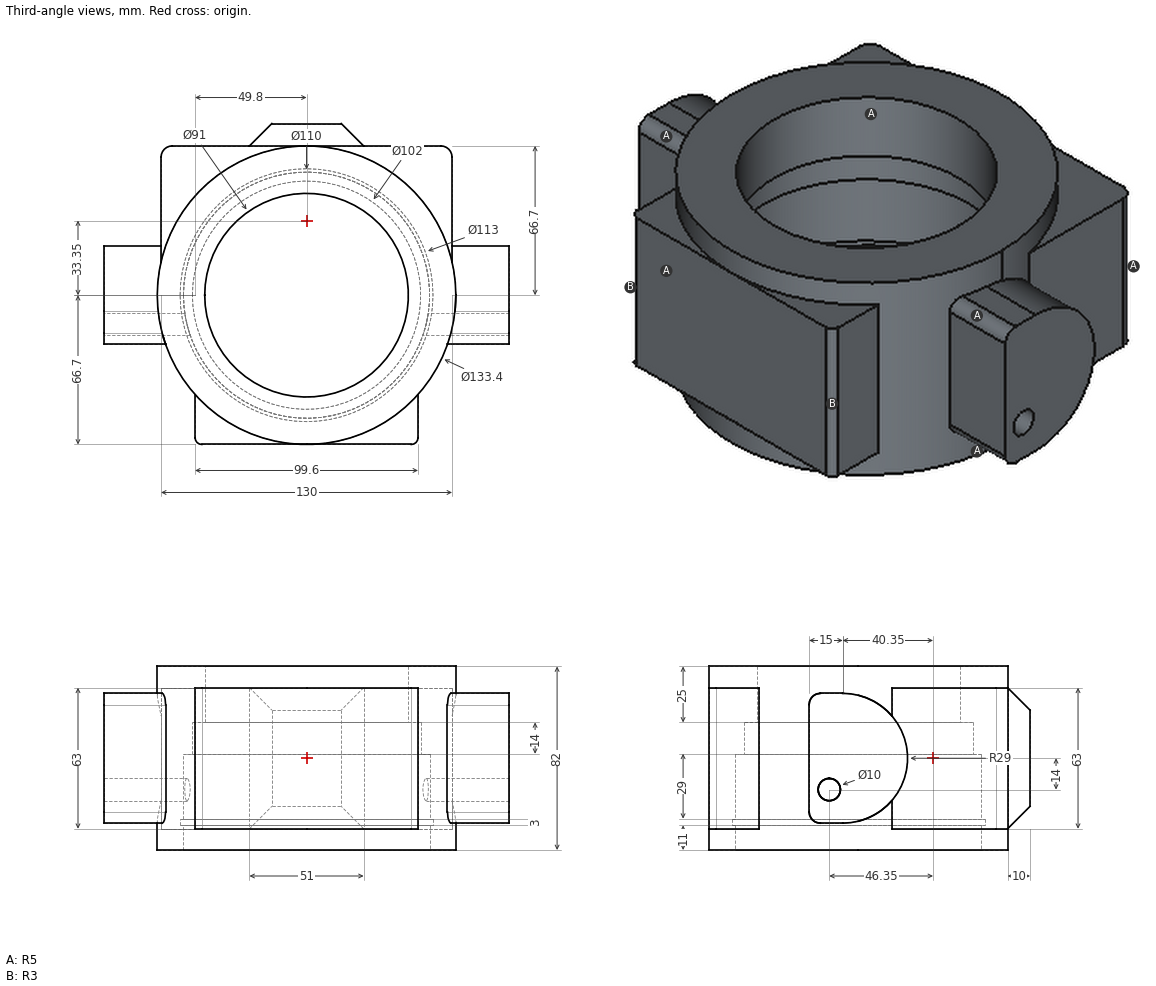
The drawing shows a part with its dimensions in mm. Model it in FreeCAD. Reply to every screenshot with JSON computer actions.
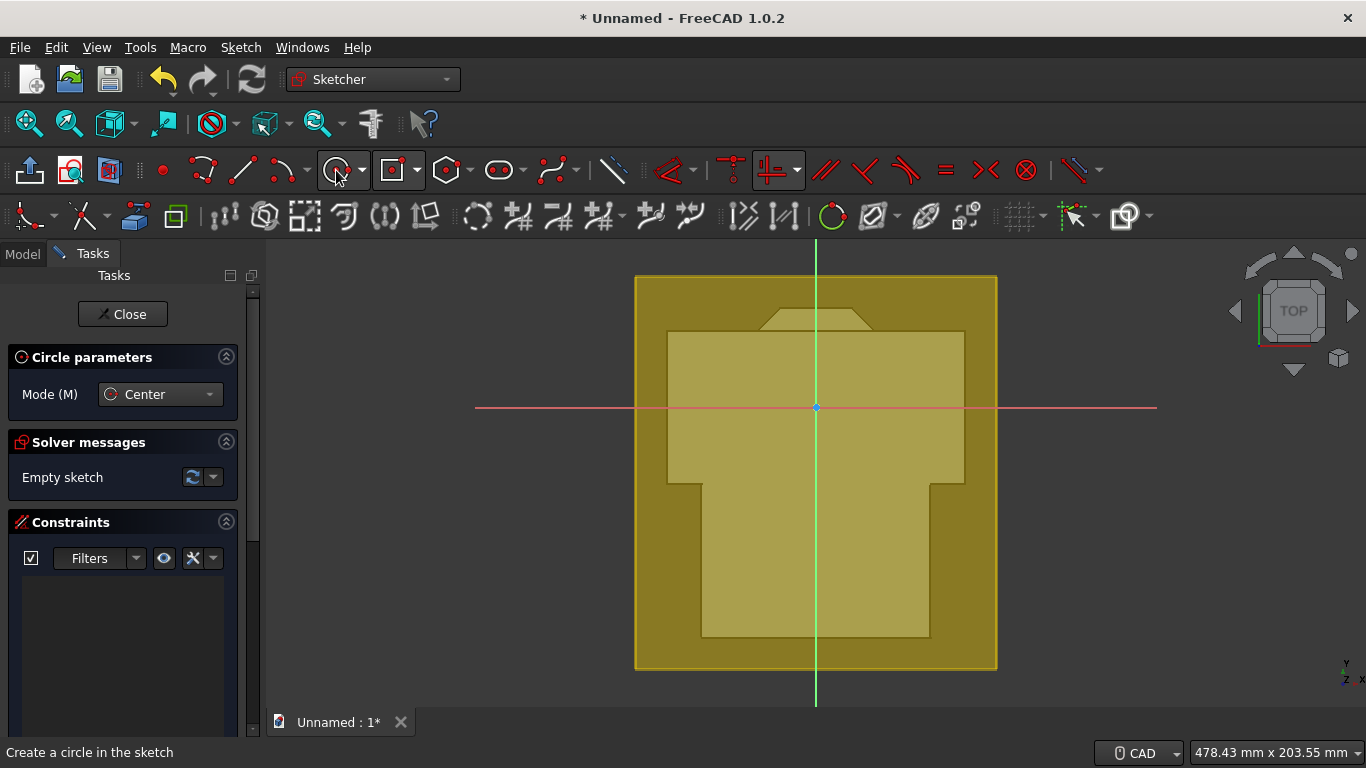
{"action": "left_click", "coordinate": [816, 484]}
{"action": "left_click", "coordinate": [924, 376]}
{"action": "key", "text": "Escape"}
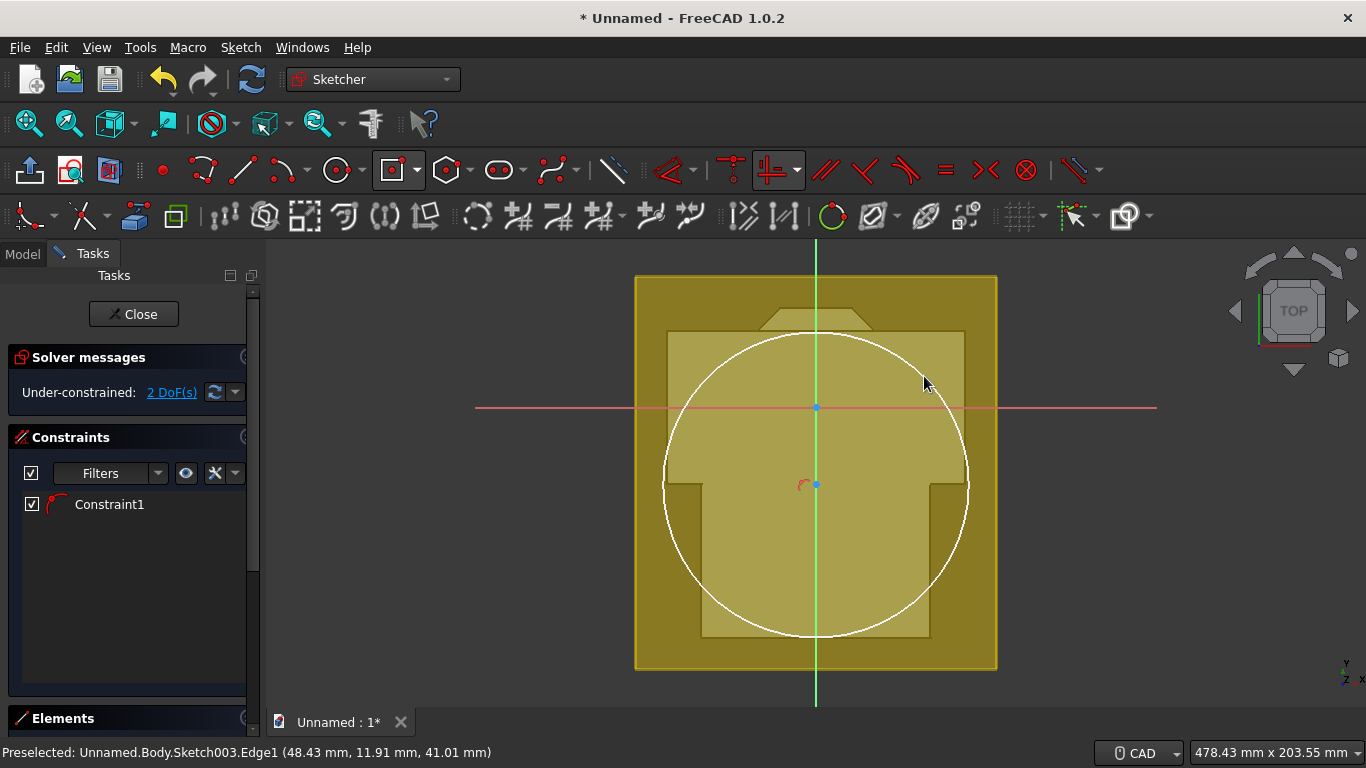
{"action": "key", "text": "d"}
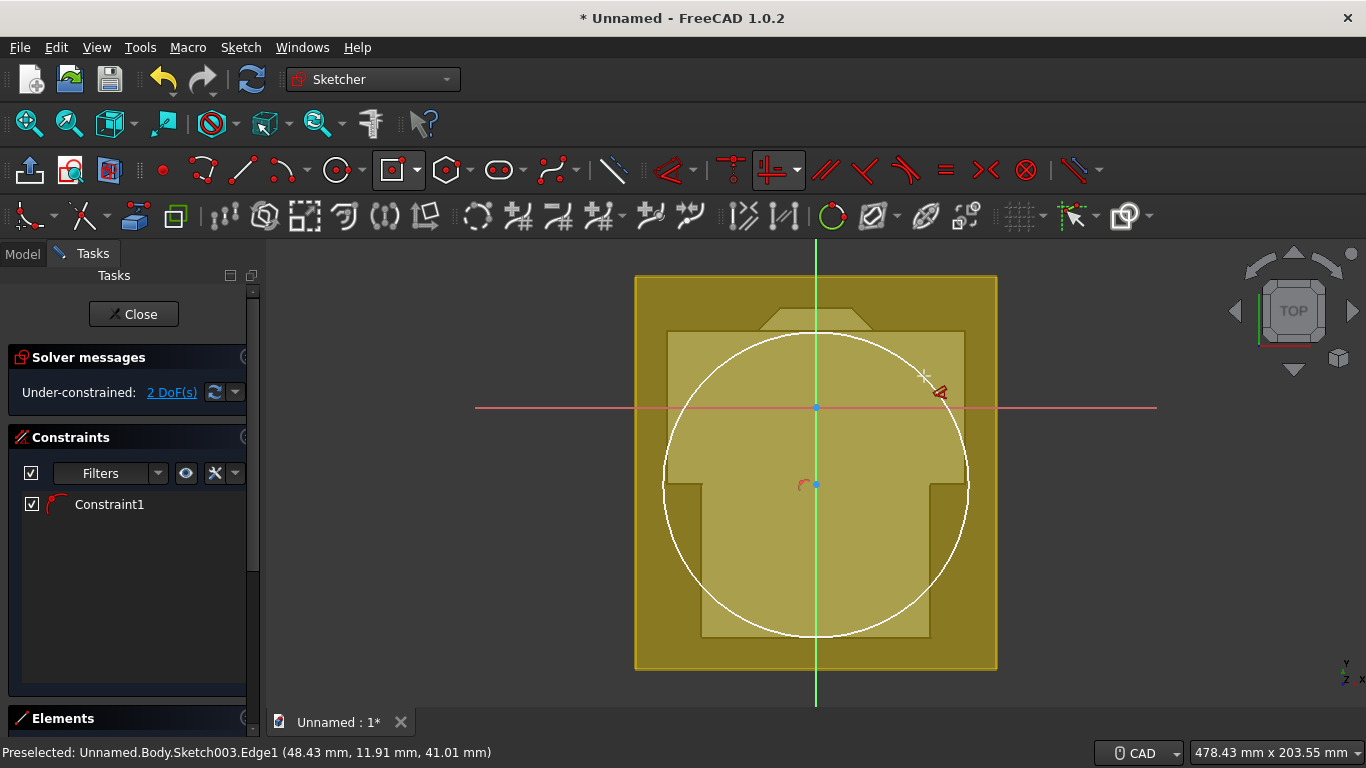
{"action": "left_click", "coordinate": [924, 377]}
{"action": "left_click", "coordinate": [947, 354]}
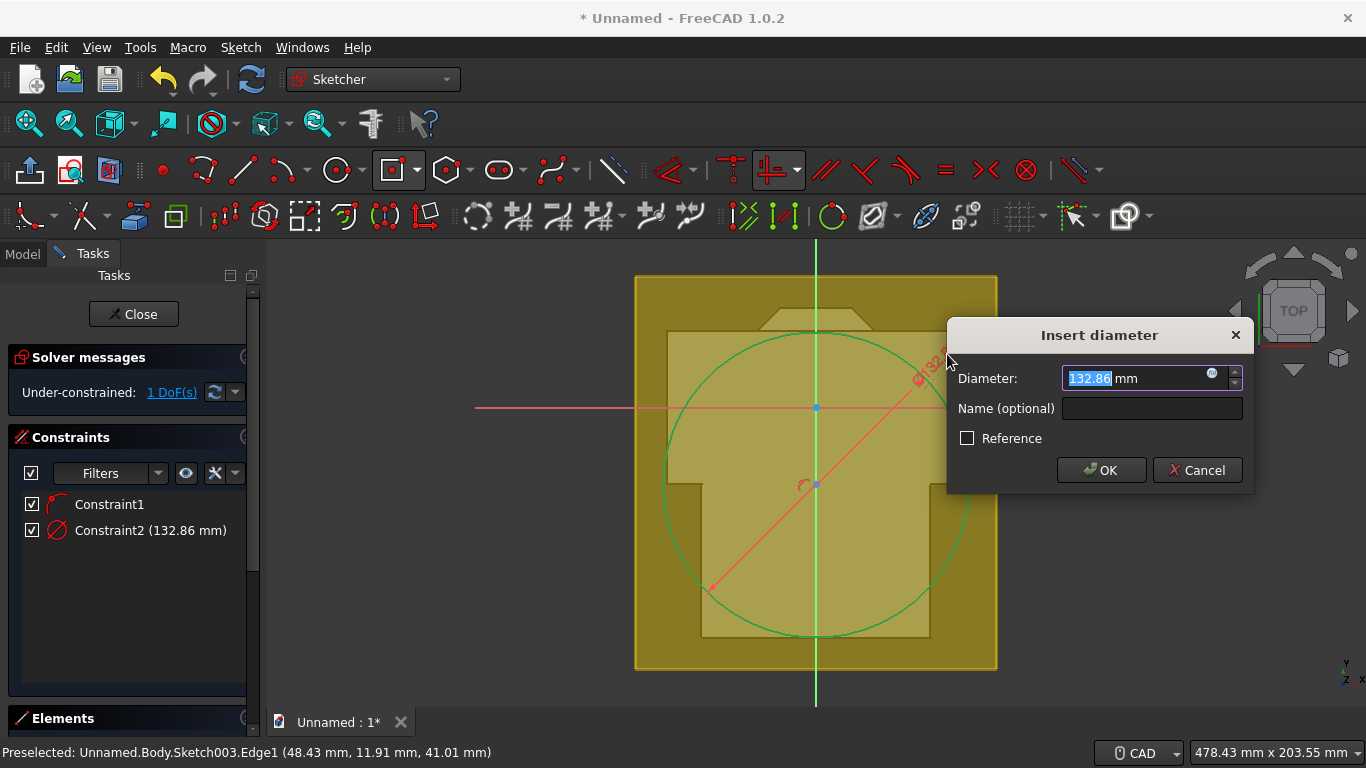
{"action": "type", "text": "133.4"}
{"action": "key", "text": "Return"}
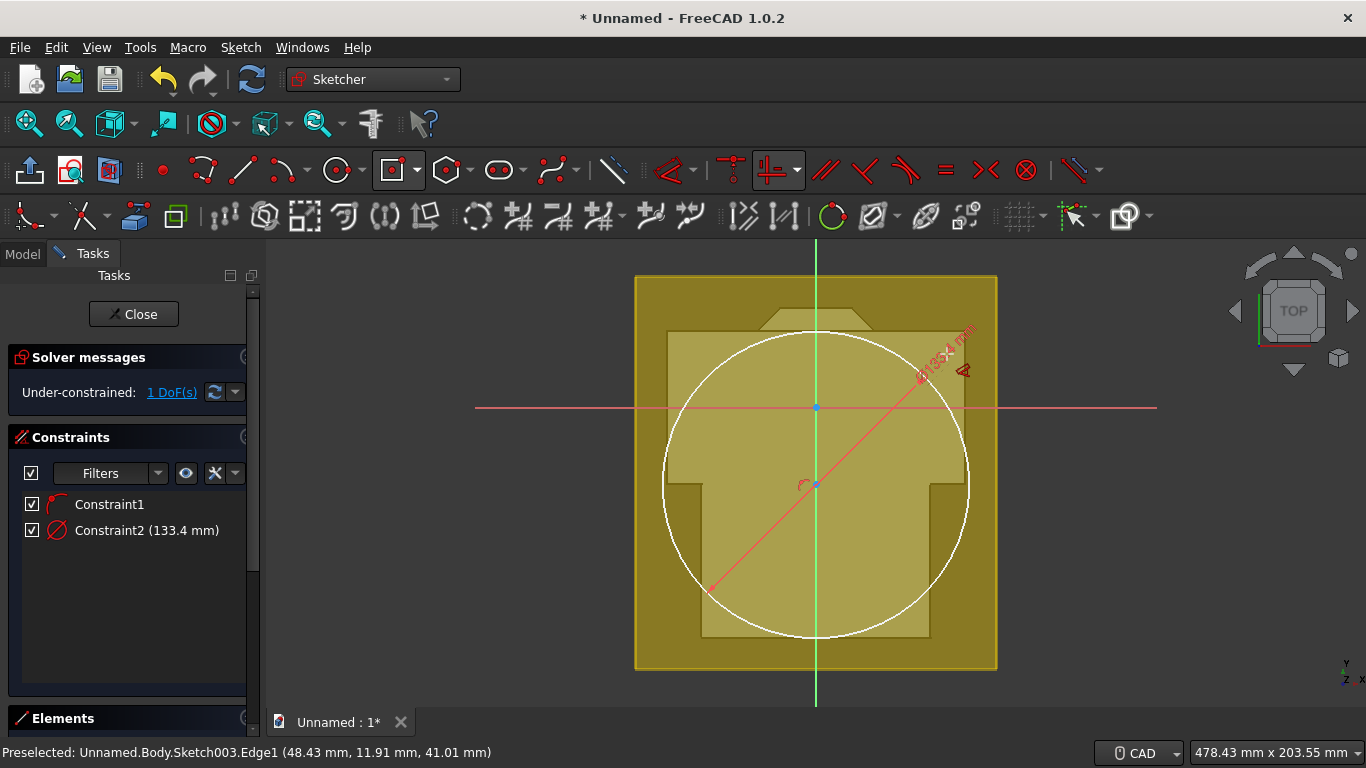
{"action": "left_click", "coordinate": [816, 485]}
{"action": "left_click", "coordinate": [850, 446]}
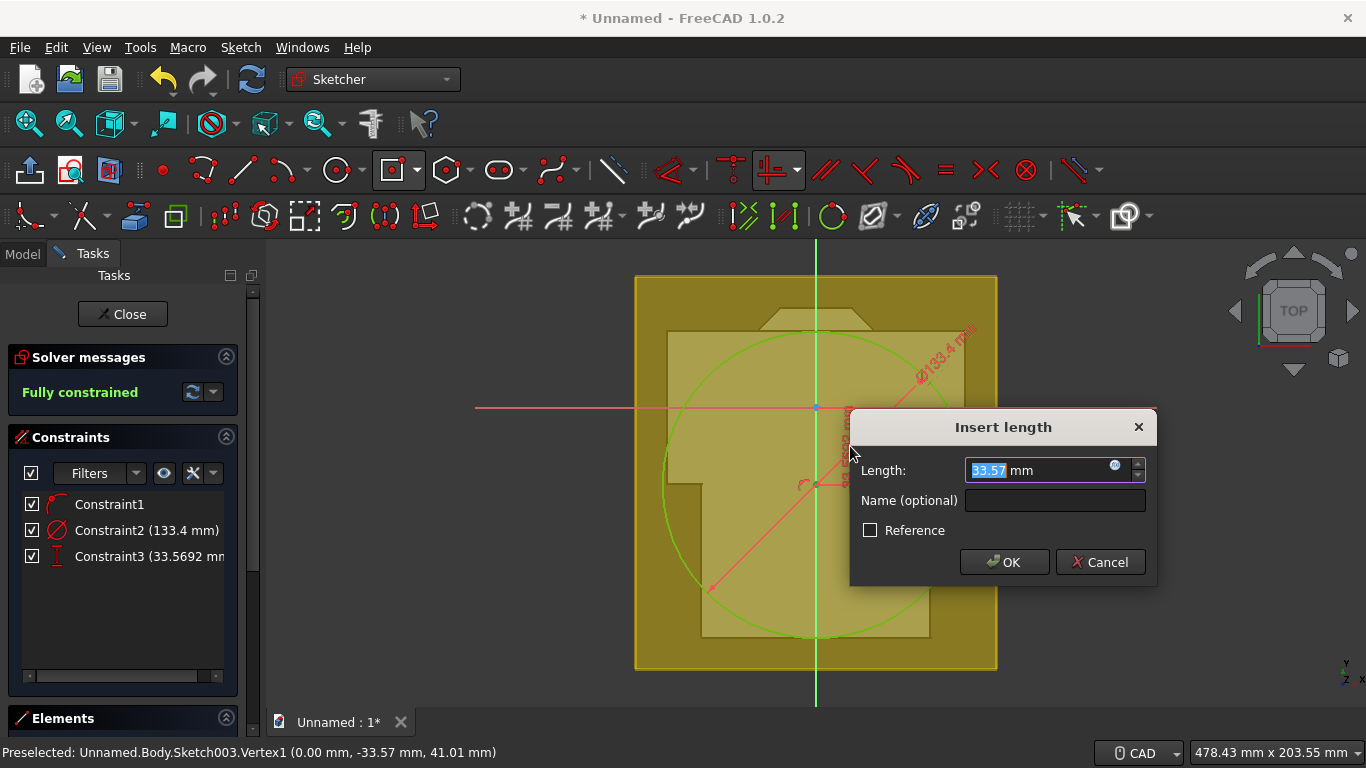
{"action": "type", "text": "33.35"}
{"action": "key", "text": "Return"}
{"action": "key", "text": "Escape"}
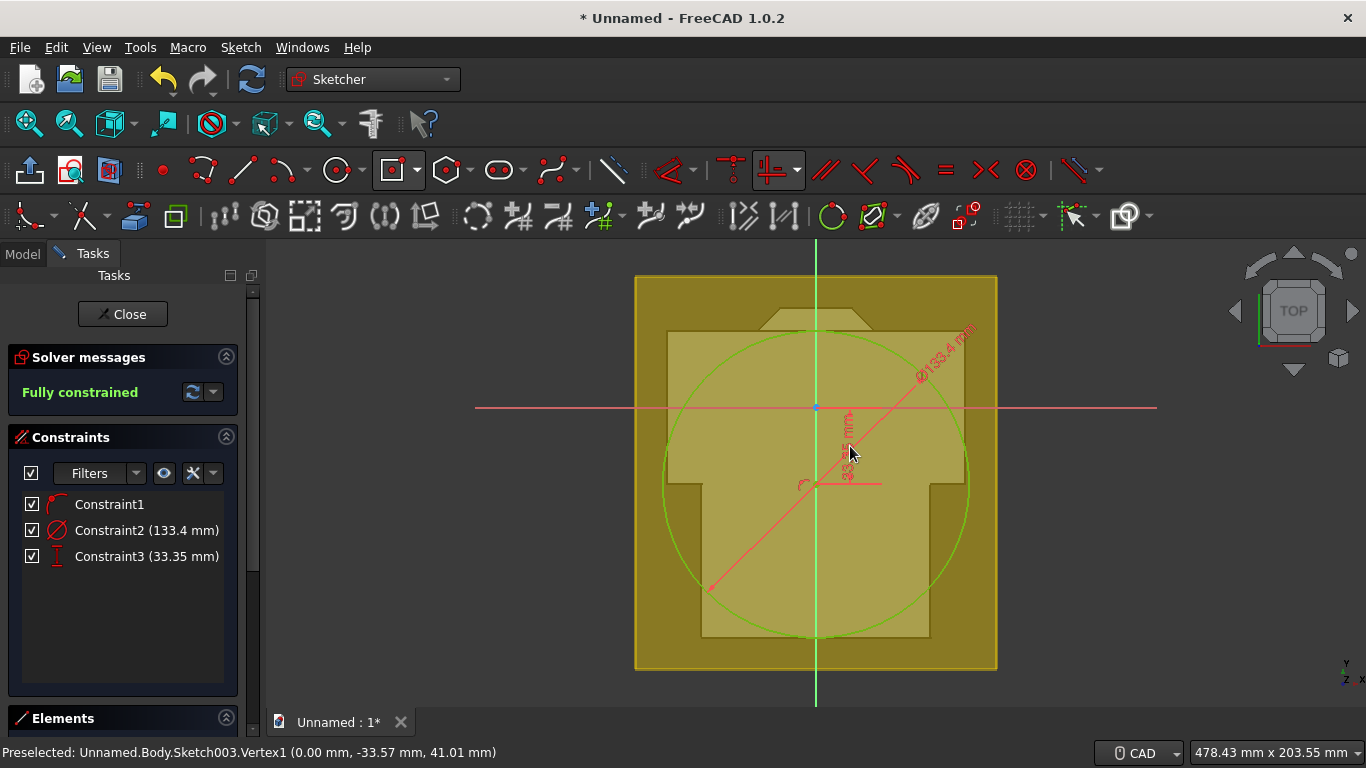
{"action": "left_click", "coordinate": [123, 314]}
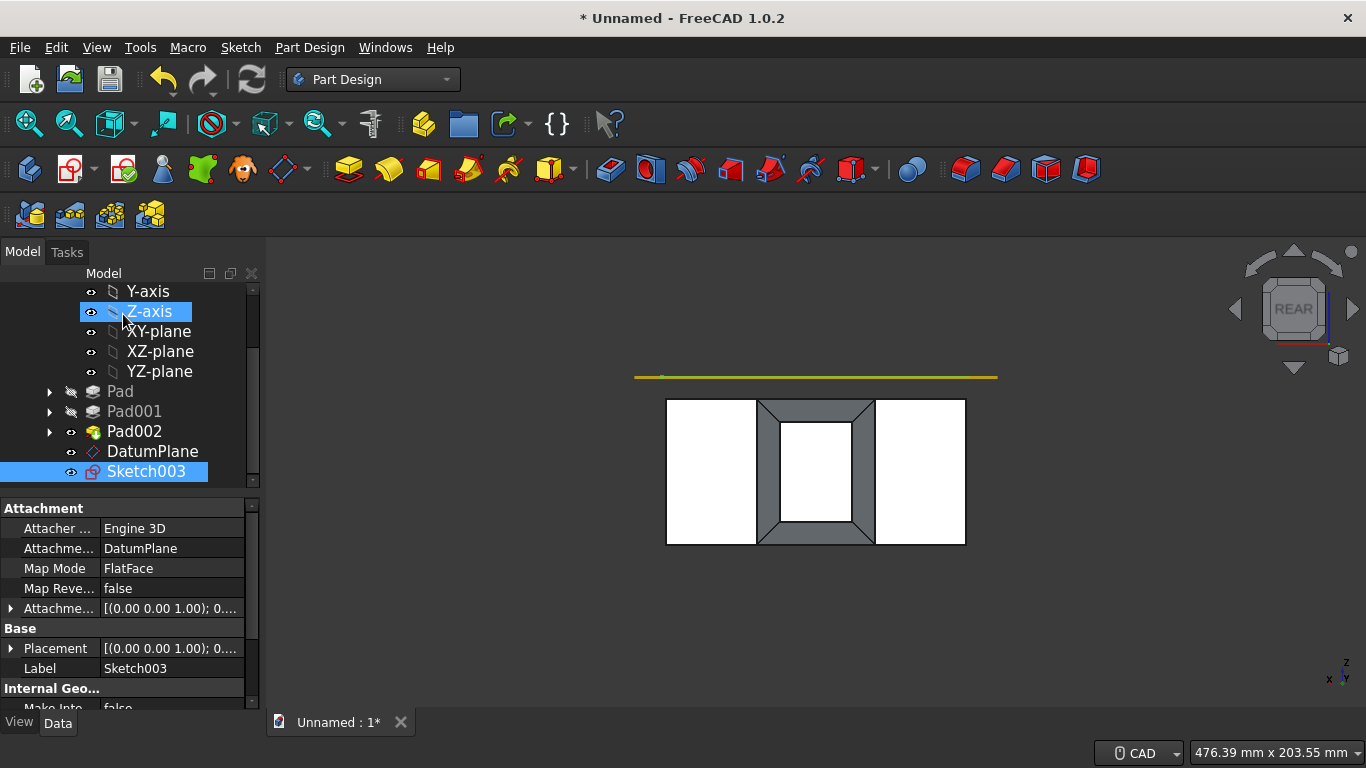
{"action": "left_click", "coordinate": [350, 170]}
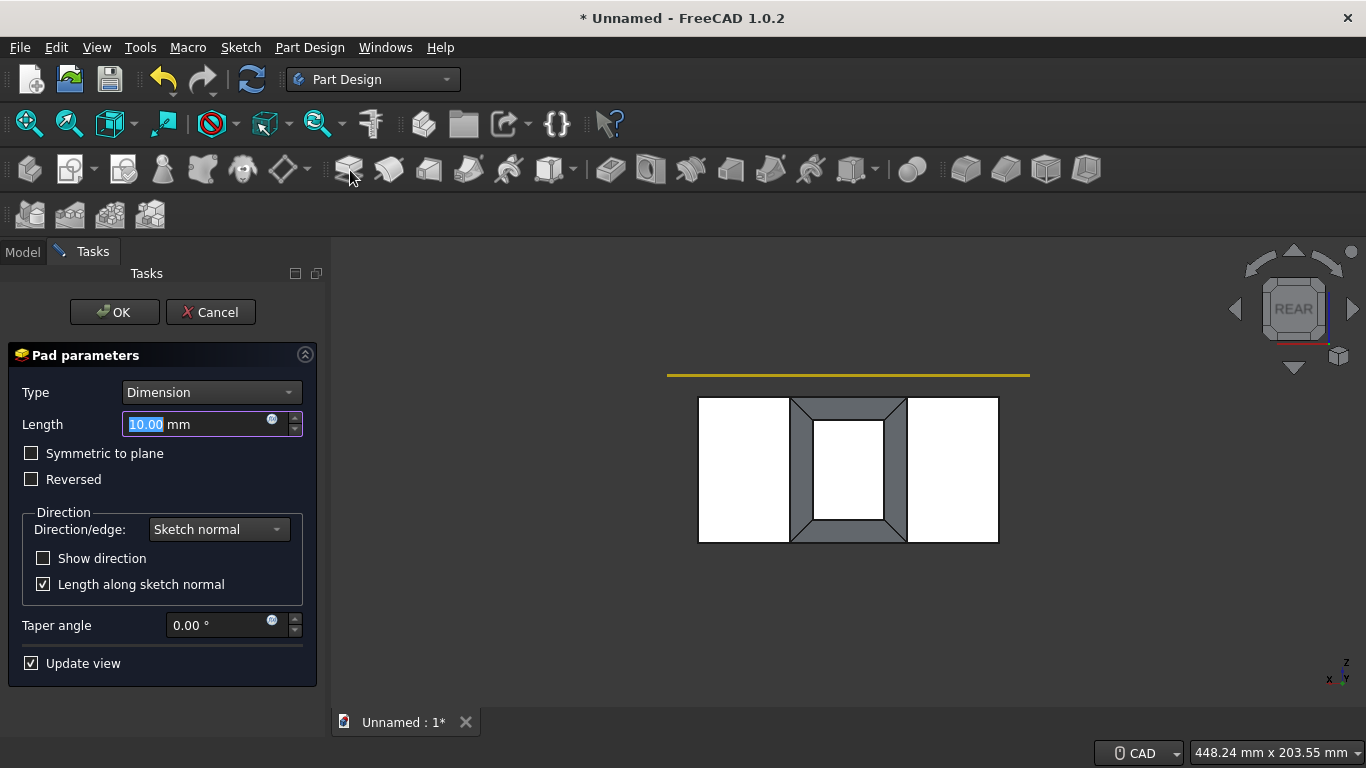
{"action": "type", "text": "82"}
{"action": "key", "text": "Tab"}